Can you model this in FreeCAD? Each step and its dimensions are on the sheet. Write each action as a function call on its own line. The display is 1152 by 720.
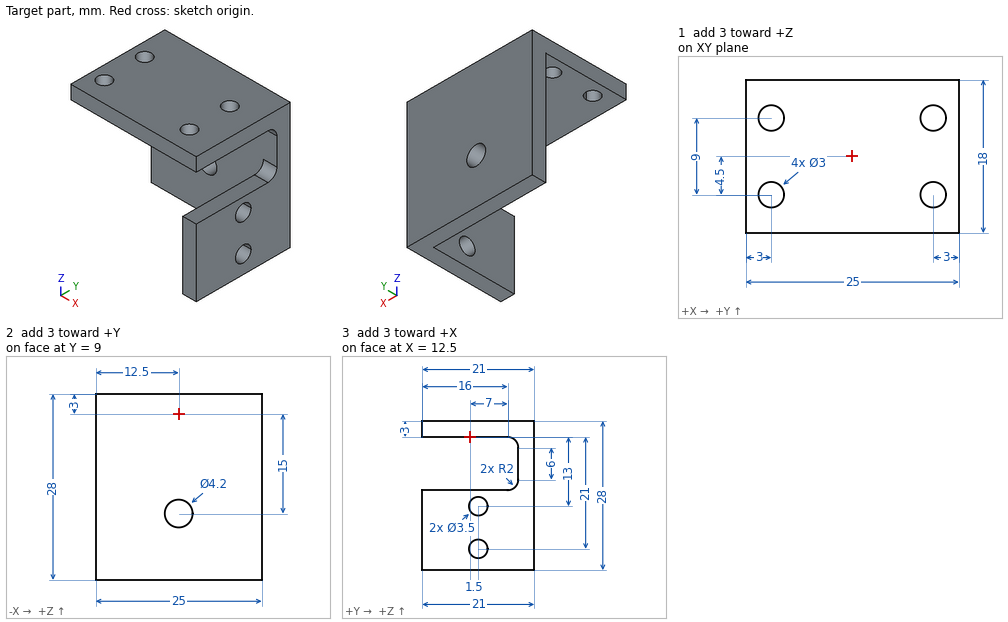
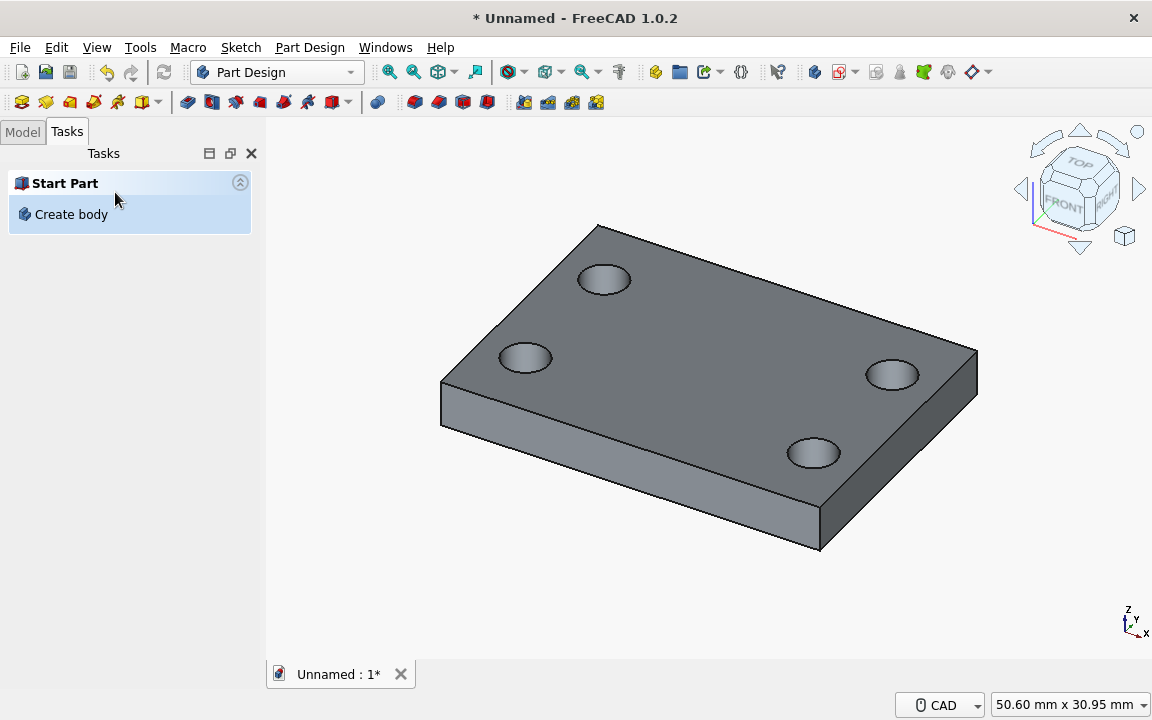
key(4)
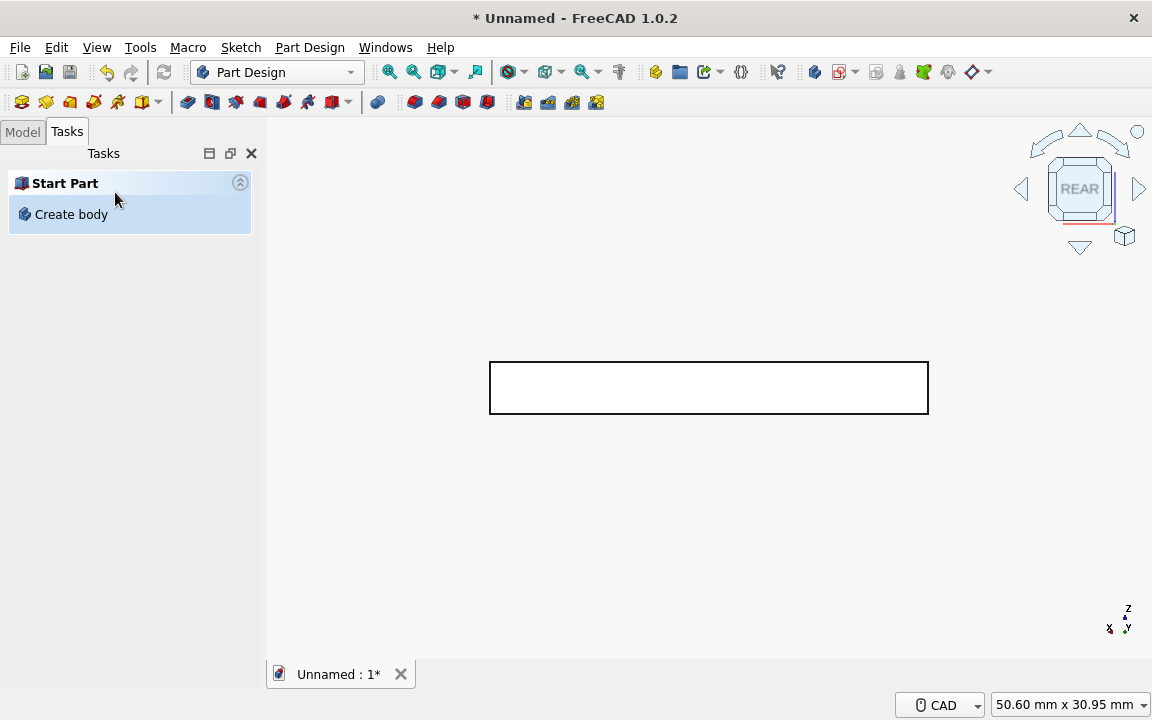
click(521, 387)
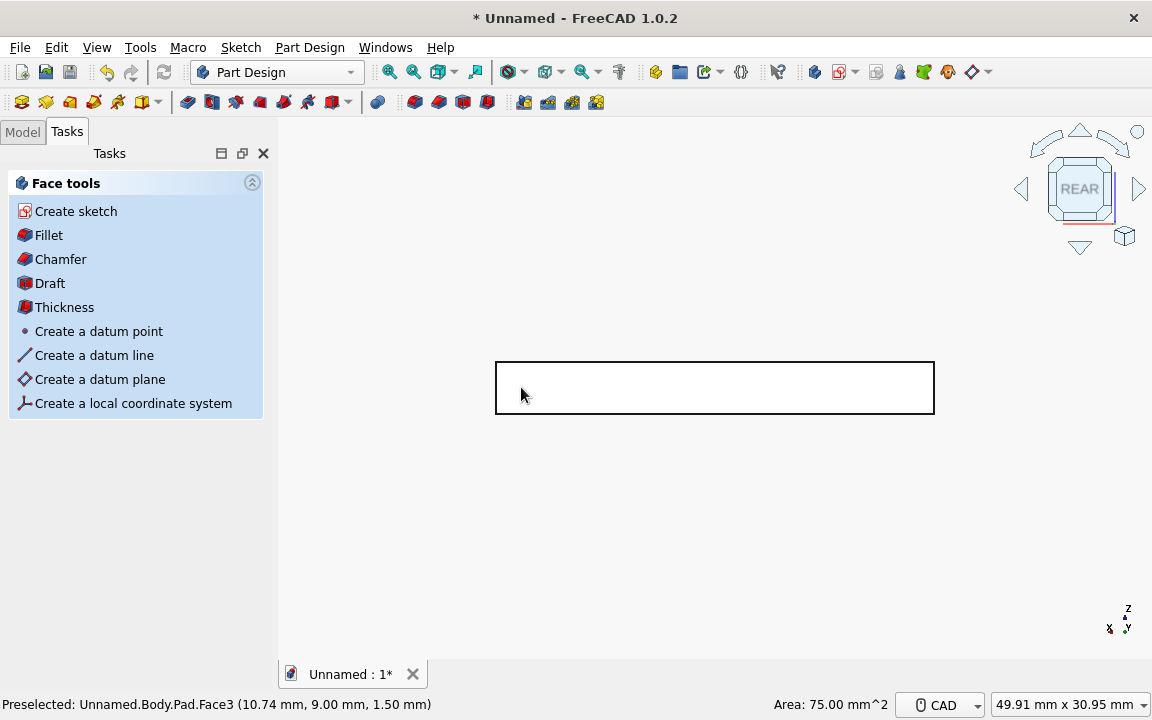
click(840, 72)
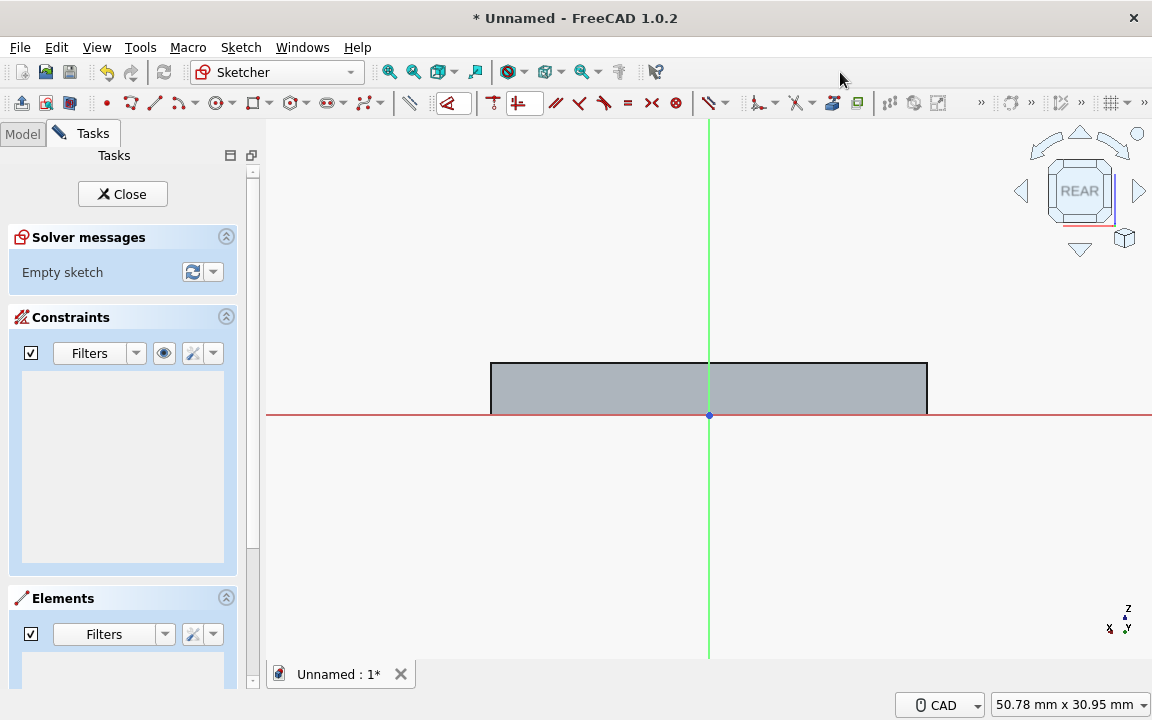
scroll(557, 147, down, 3)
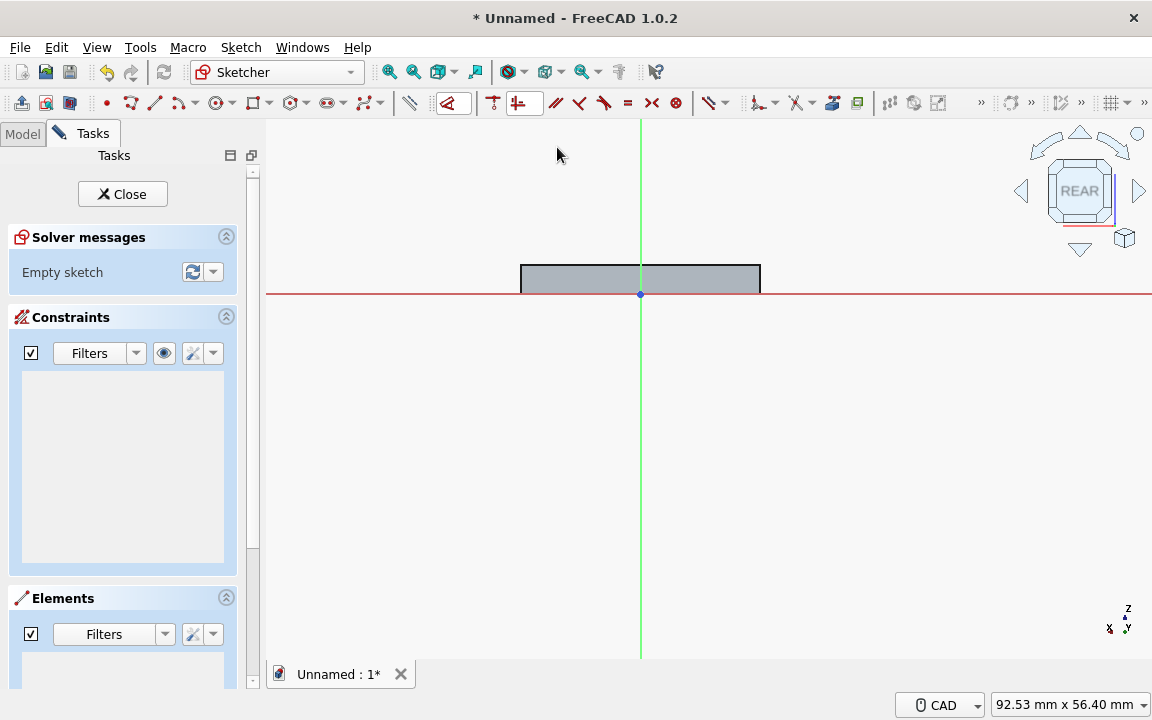
key(g)
key(r)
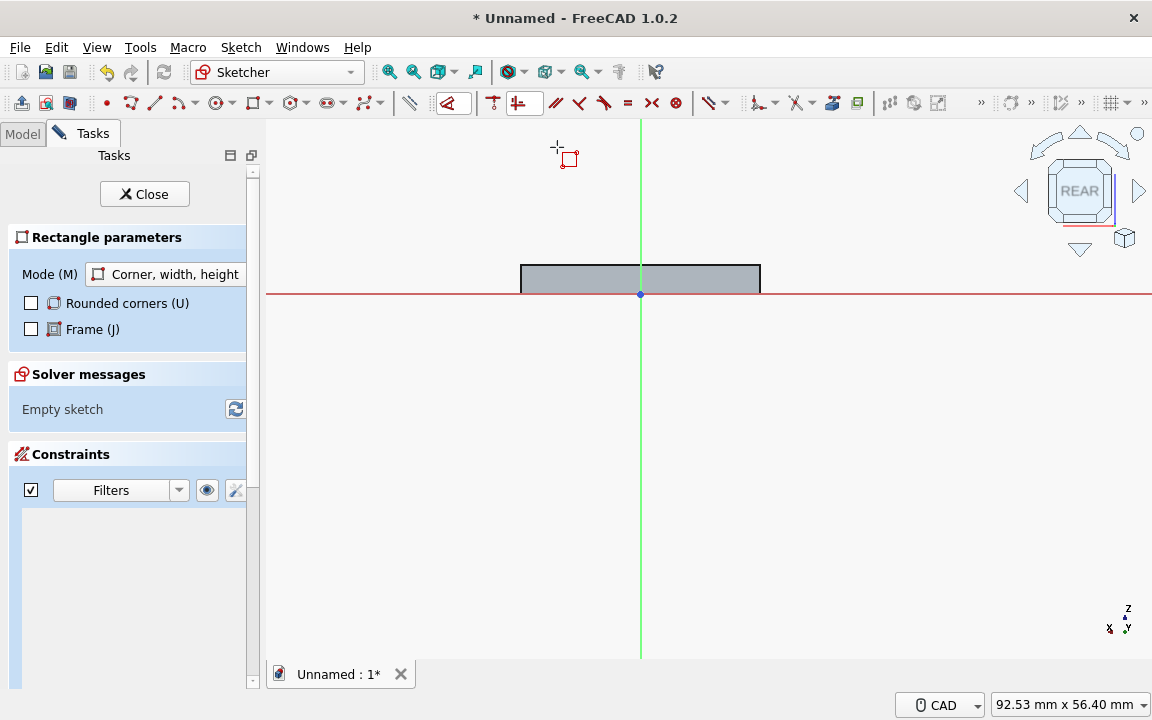
click(521, 265)
click(760, 534)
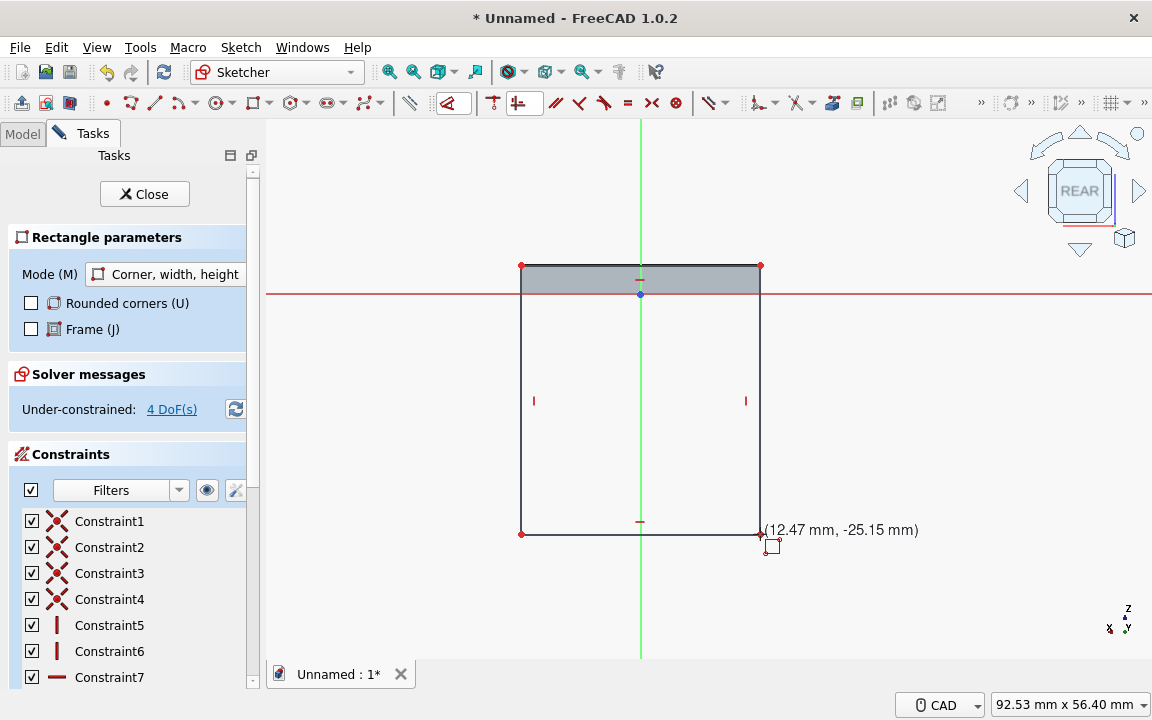
key(g)
key(c)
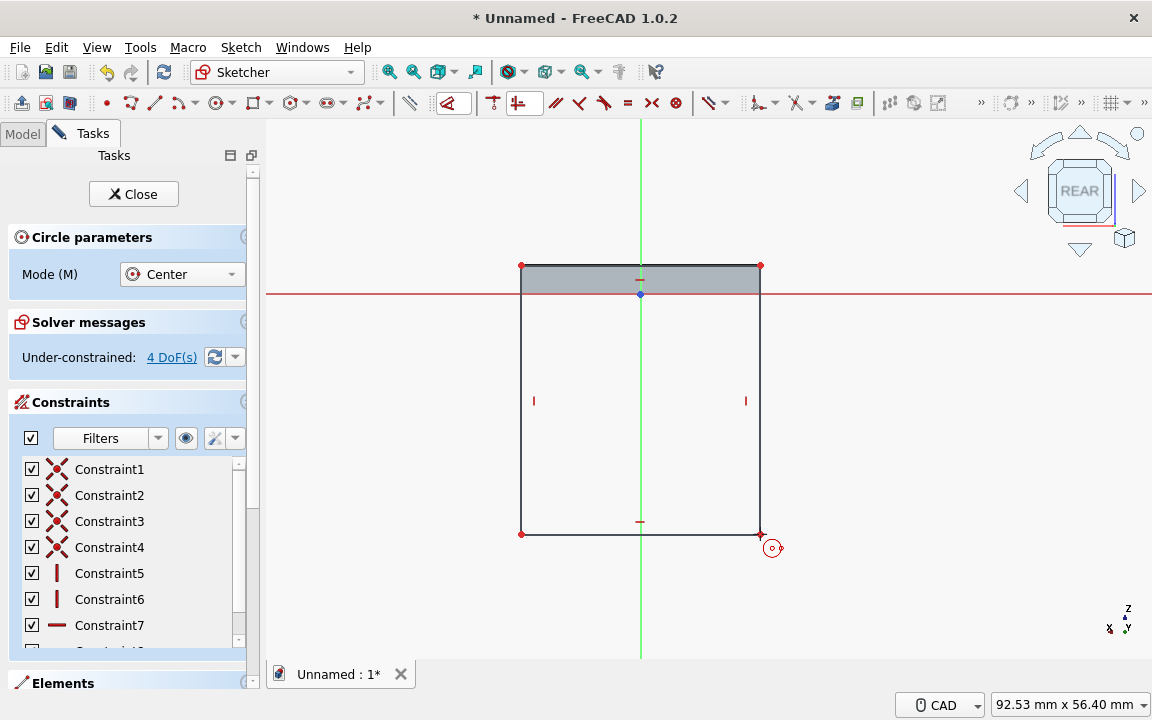
click(641, 438)
click(655, 424)
key(Escape)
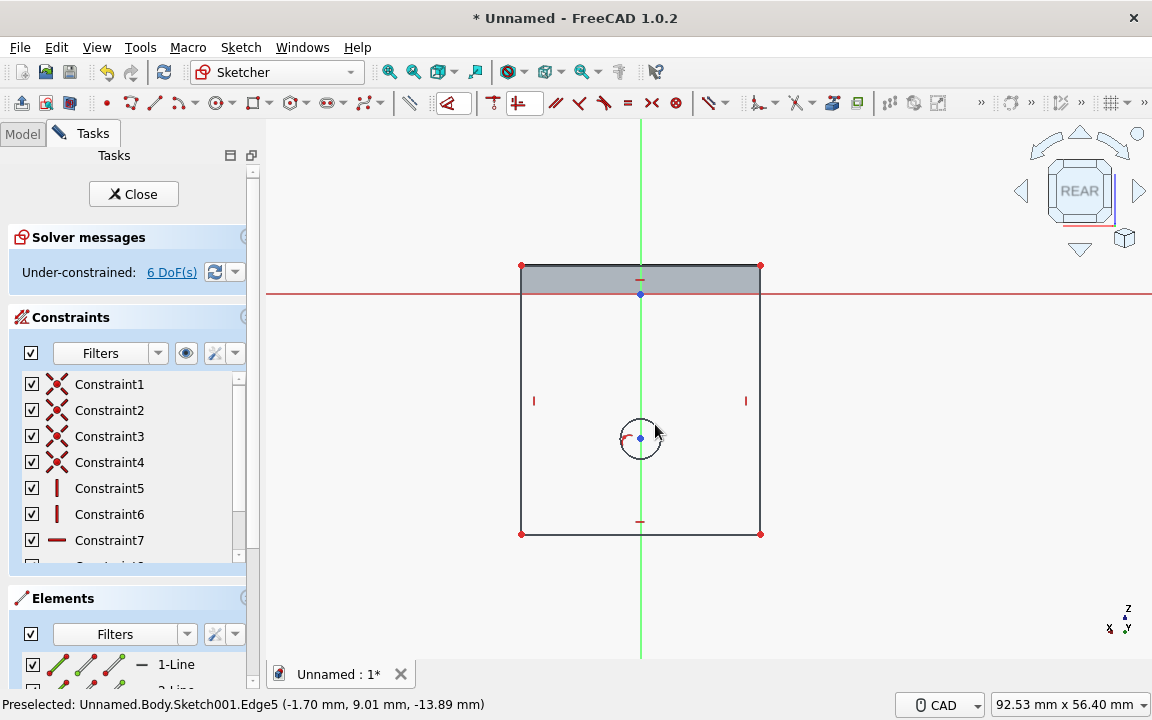
click(655, 425)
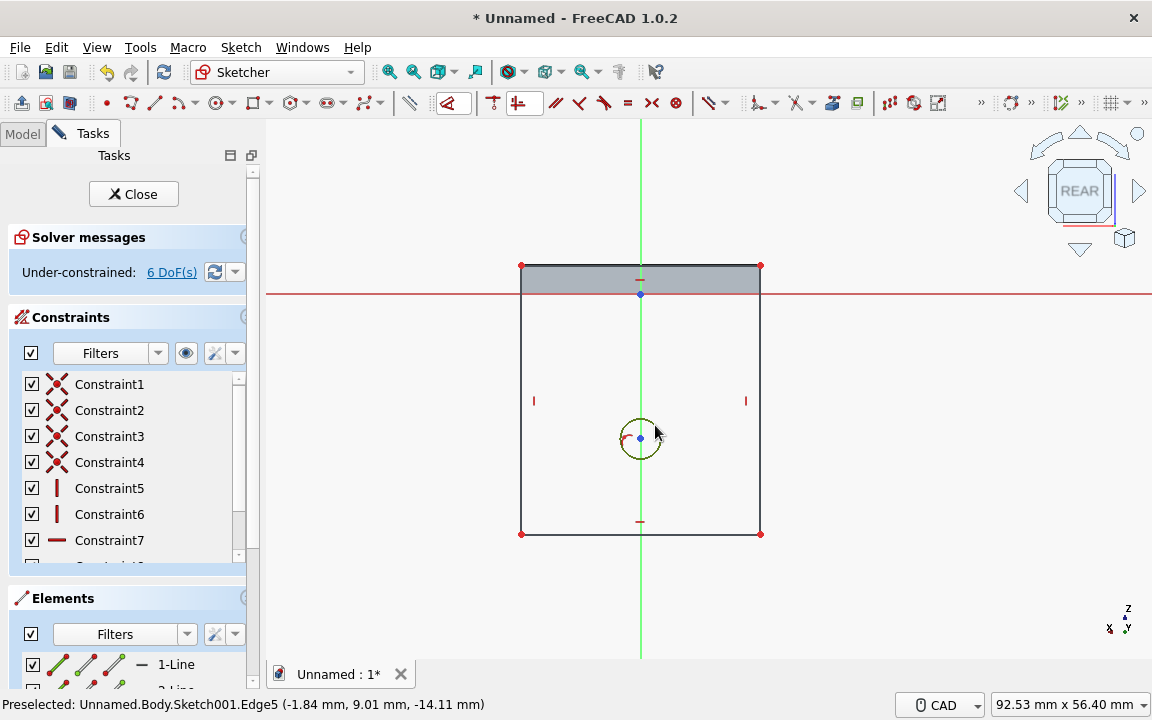
key(k)
key(o)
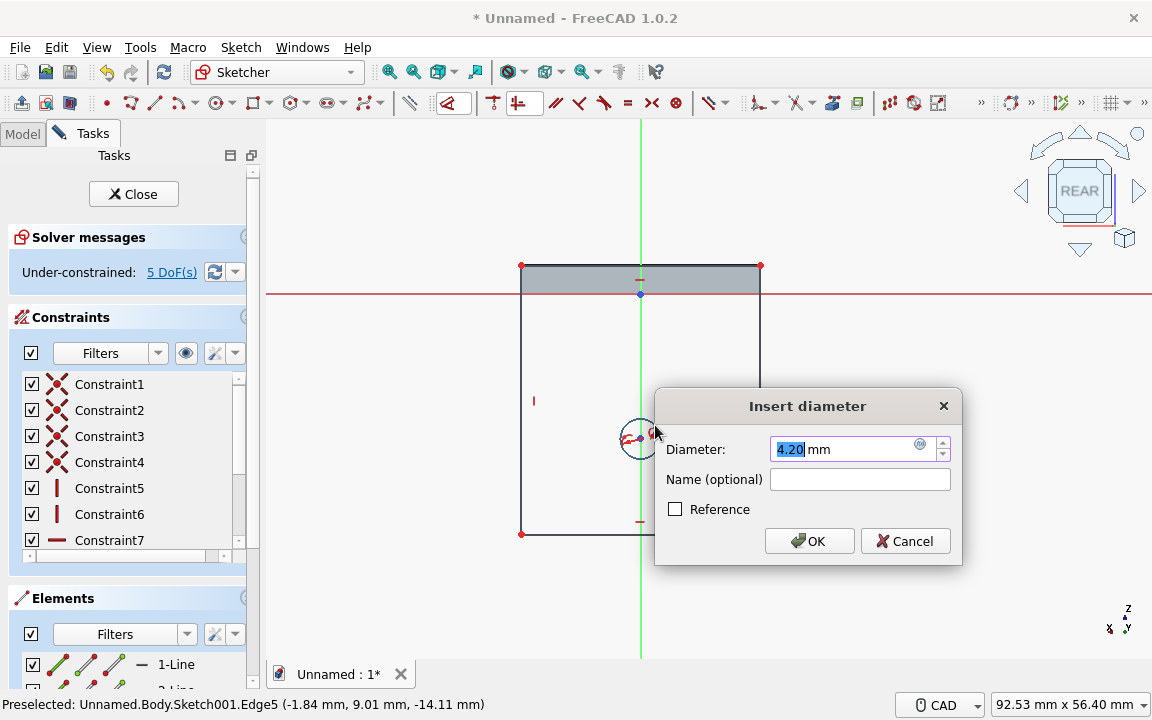
text(4.2)
key(Return)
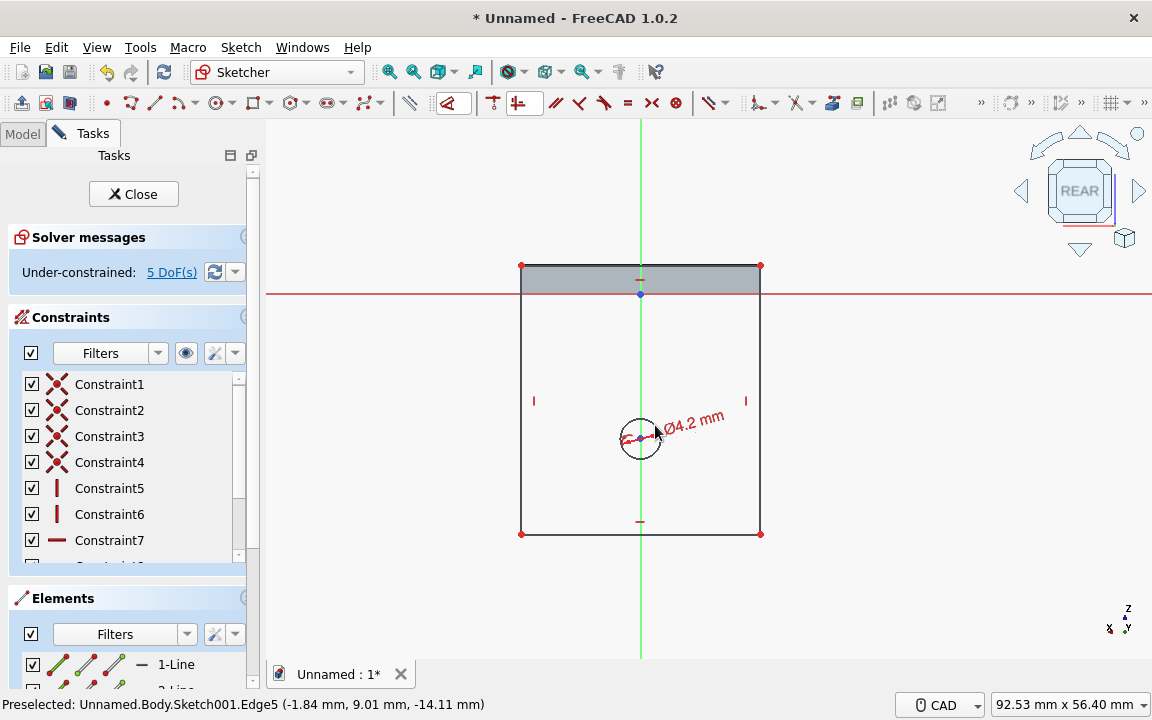
click(521, 347)